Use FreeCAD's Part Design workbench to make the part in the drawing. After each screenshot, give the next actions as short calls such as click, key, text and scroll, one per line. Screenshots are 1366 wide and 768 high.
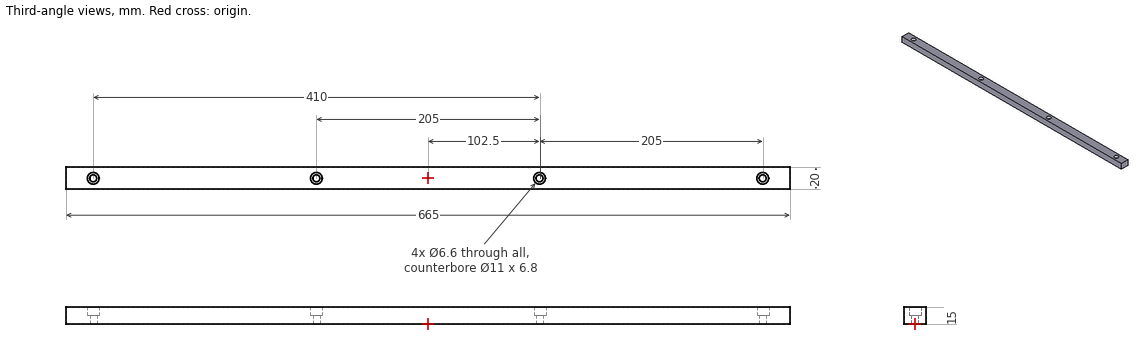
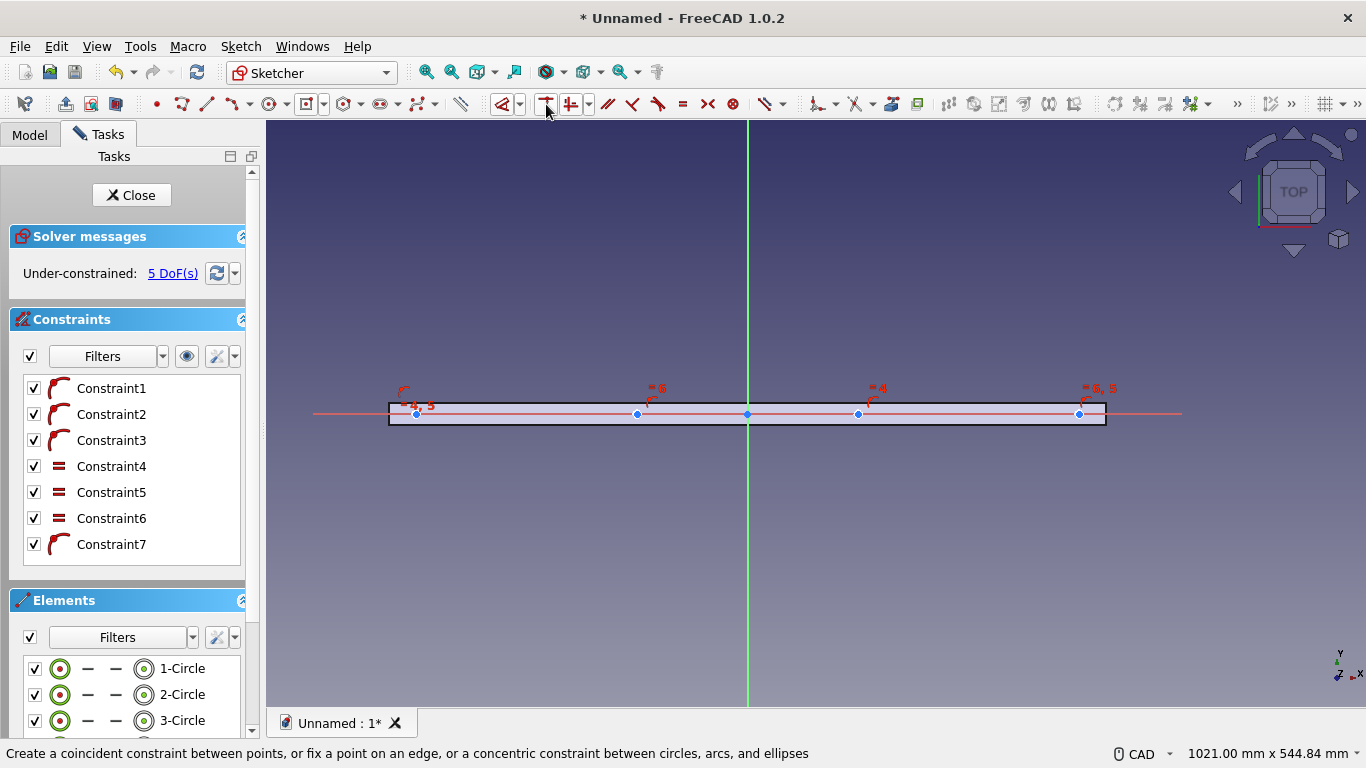
scroll(854, 414, up, 9)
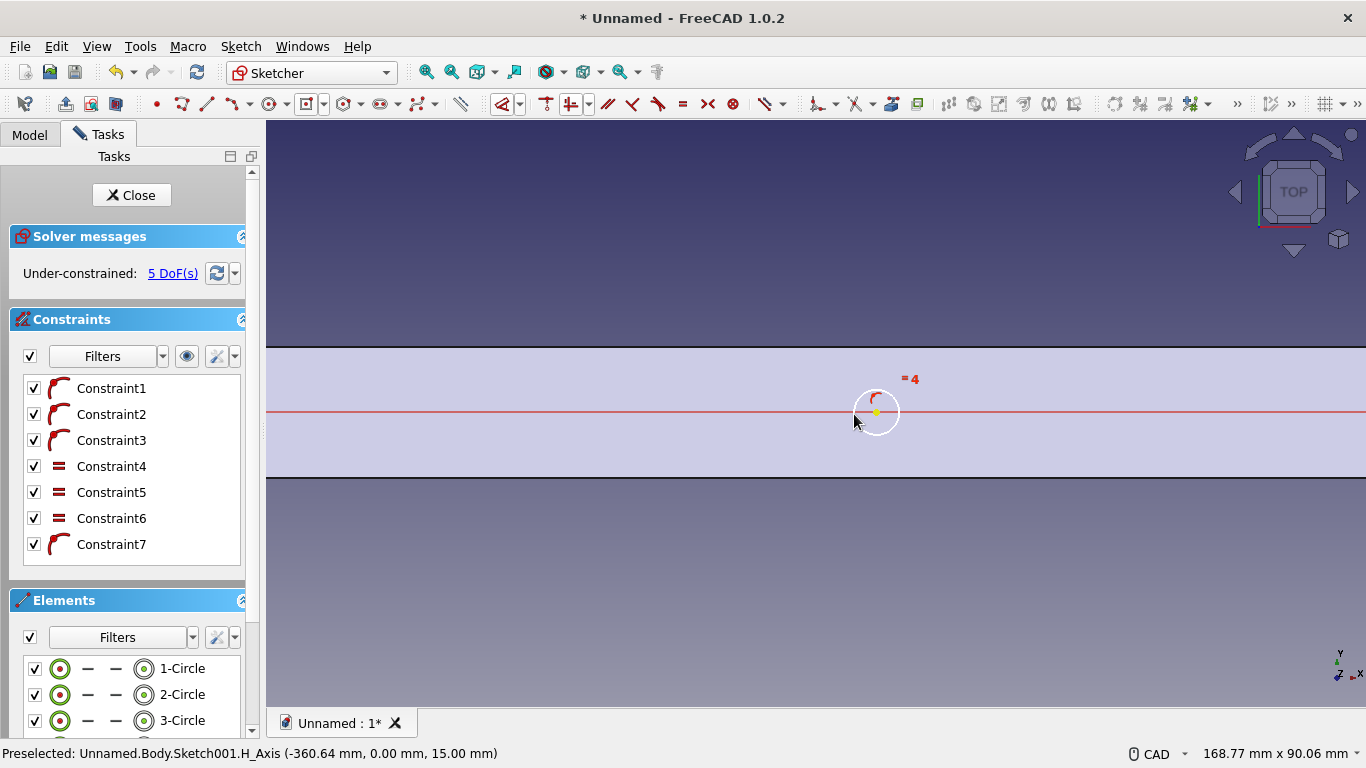
click(854, 412)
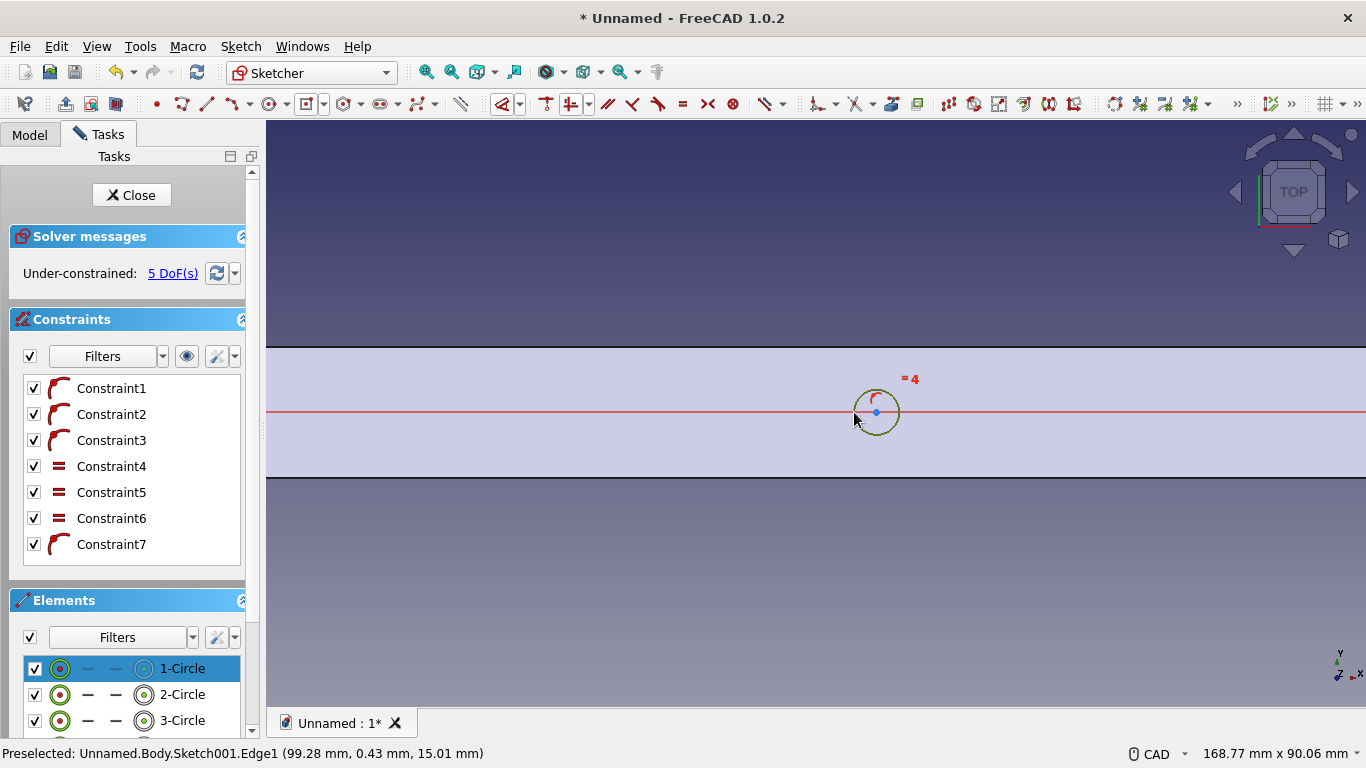
click(520, 104)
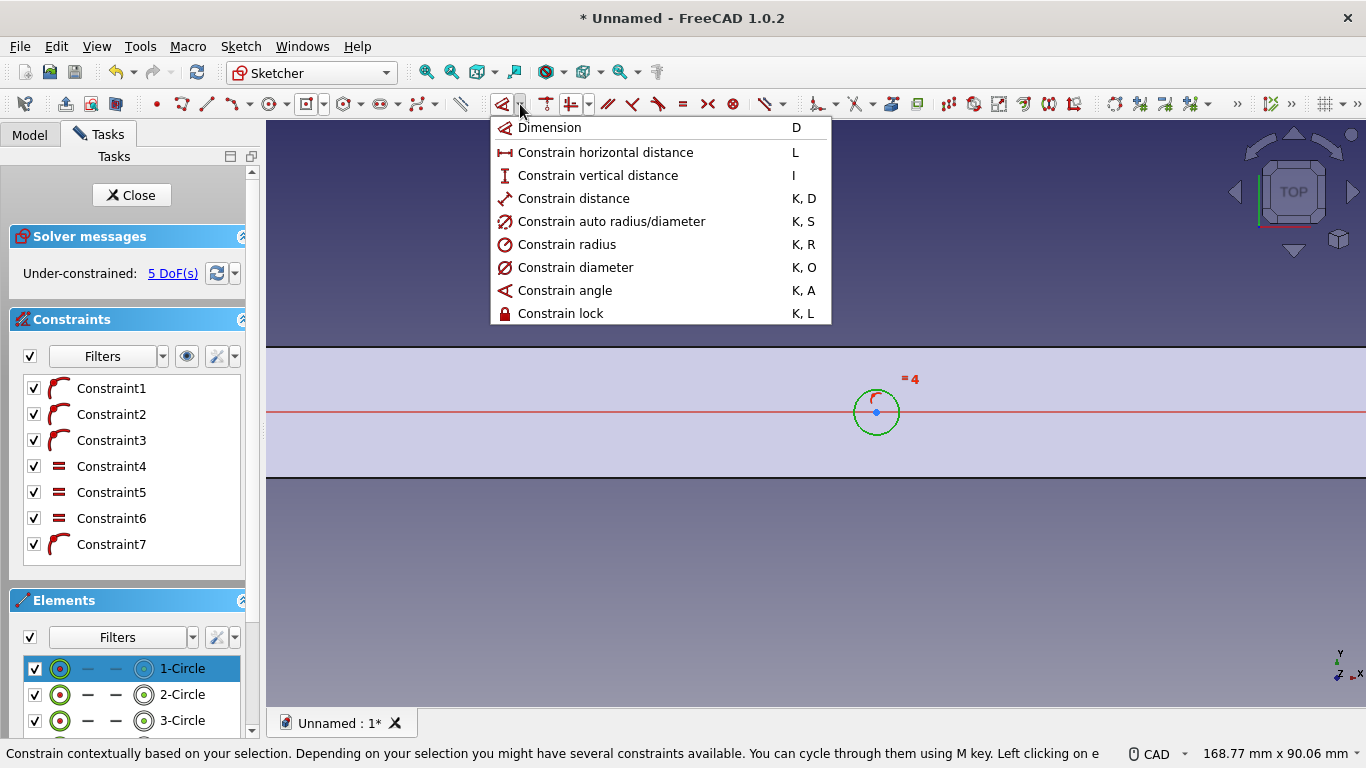
click(661, 268)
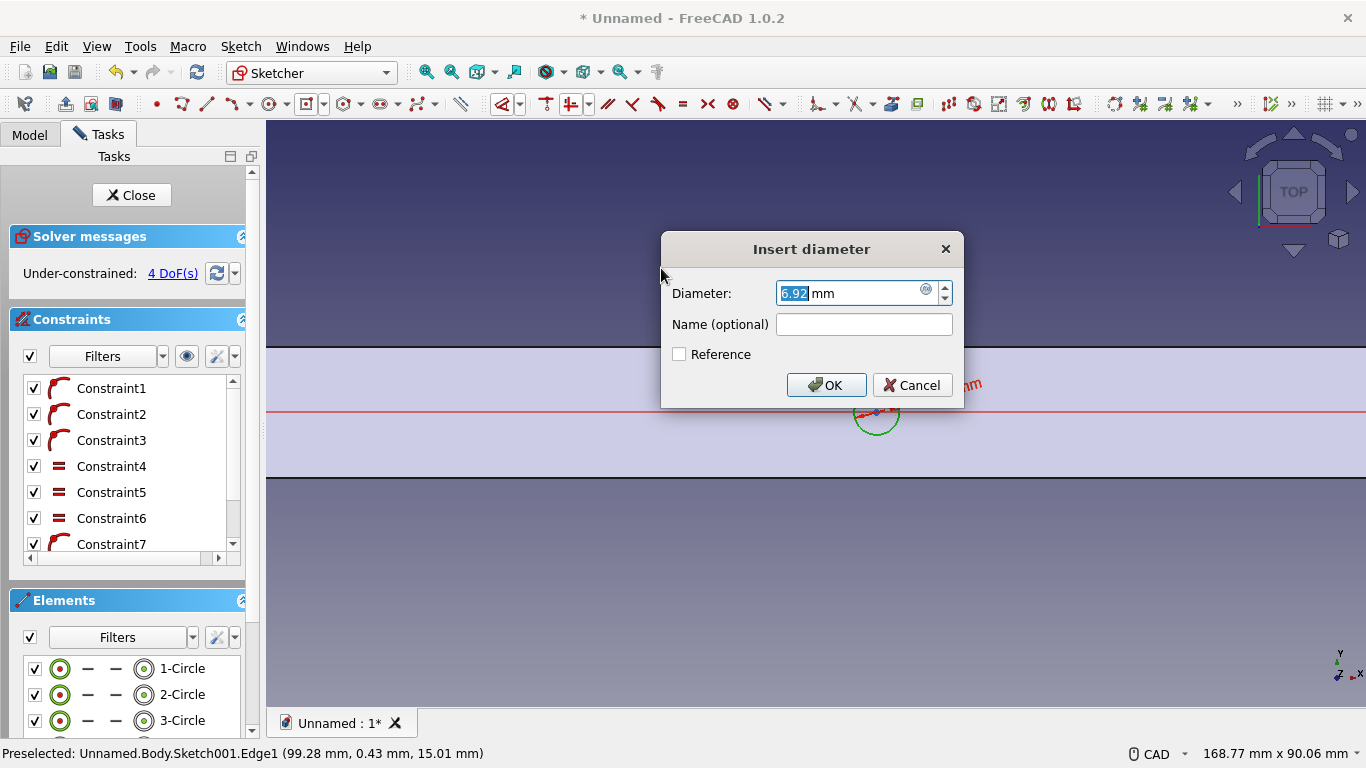
text(6.6)
key(Return)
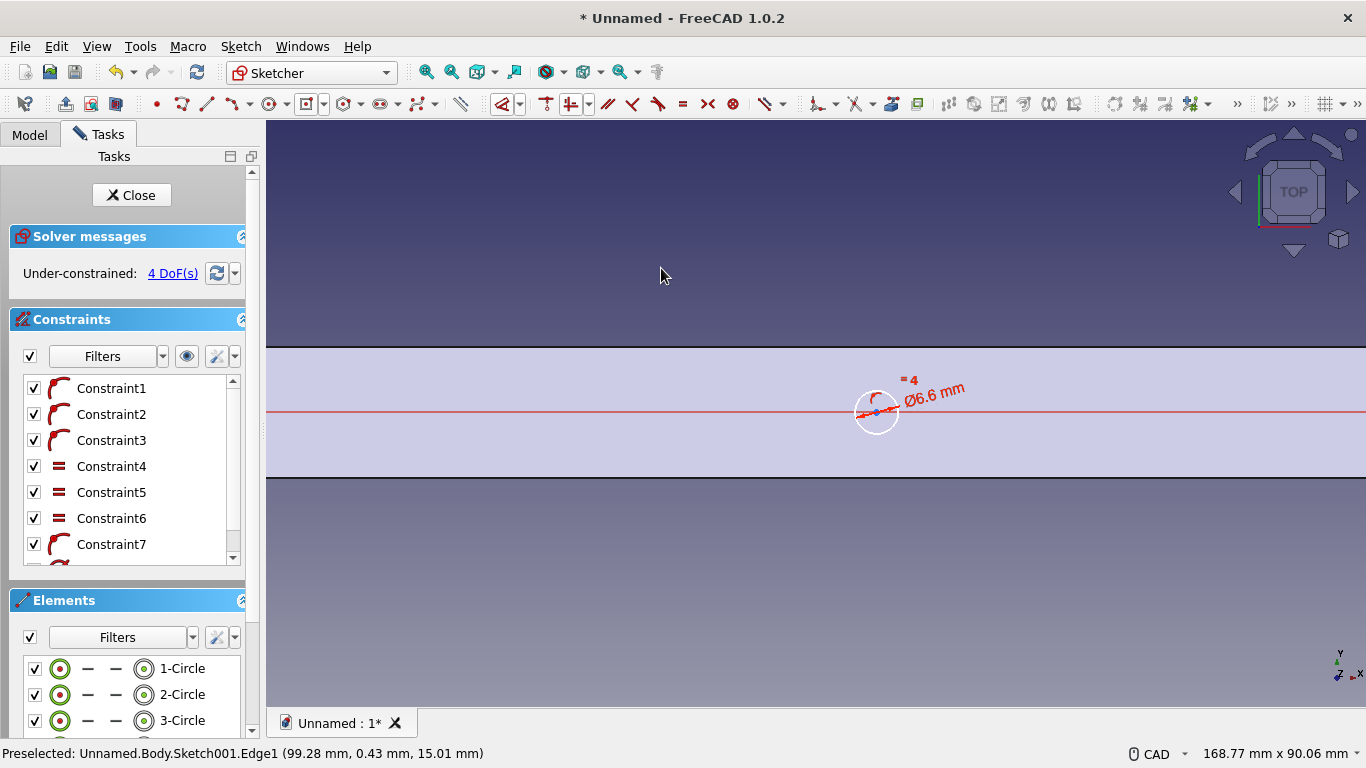
scroll(854, 414, down, 9)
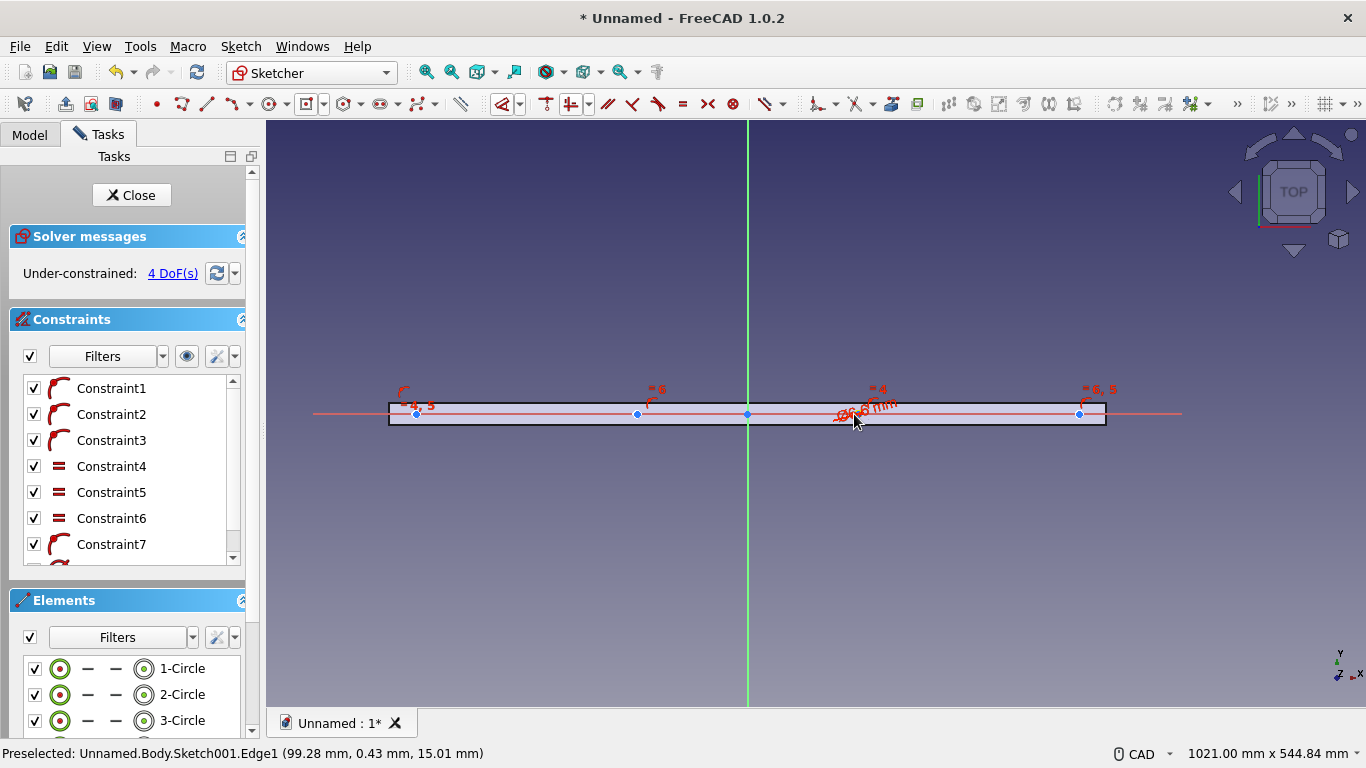
click(858, 414)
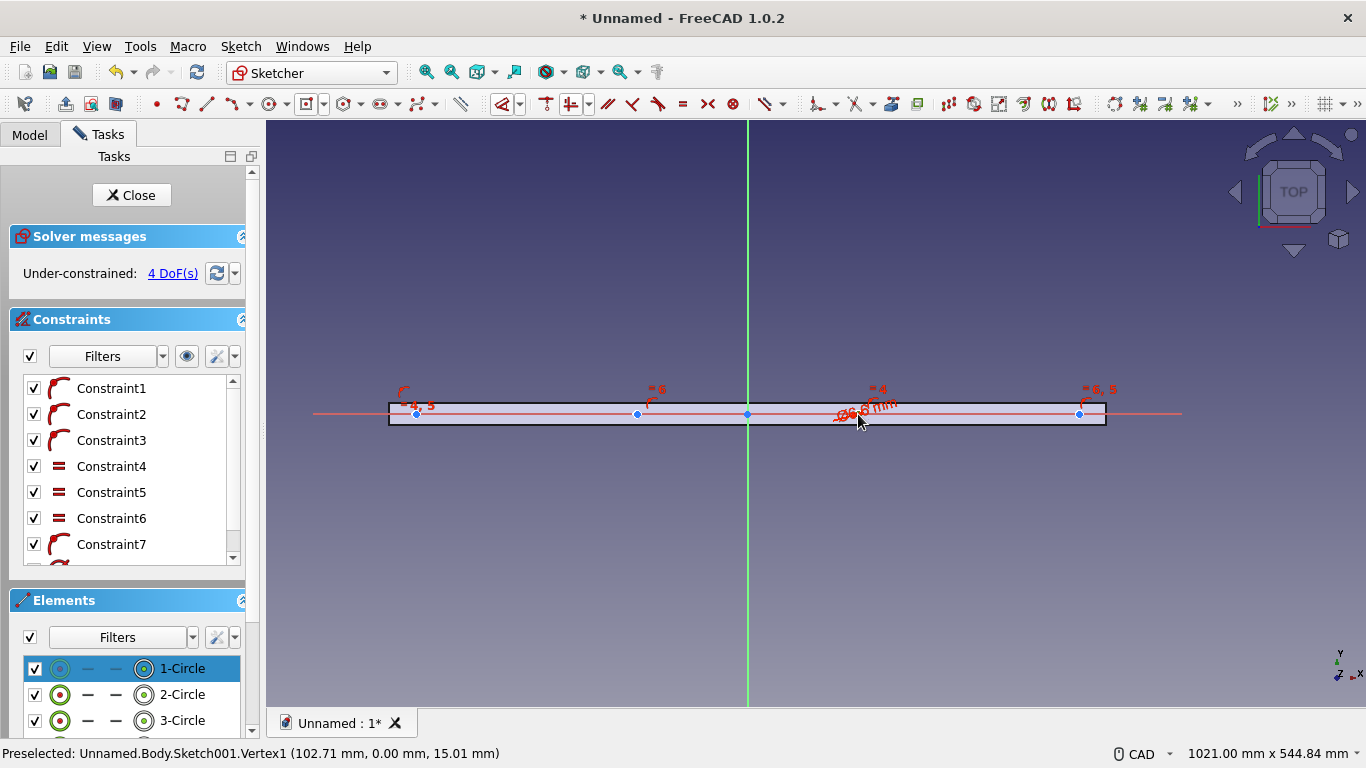
click(416, 414)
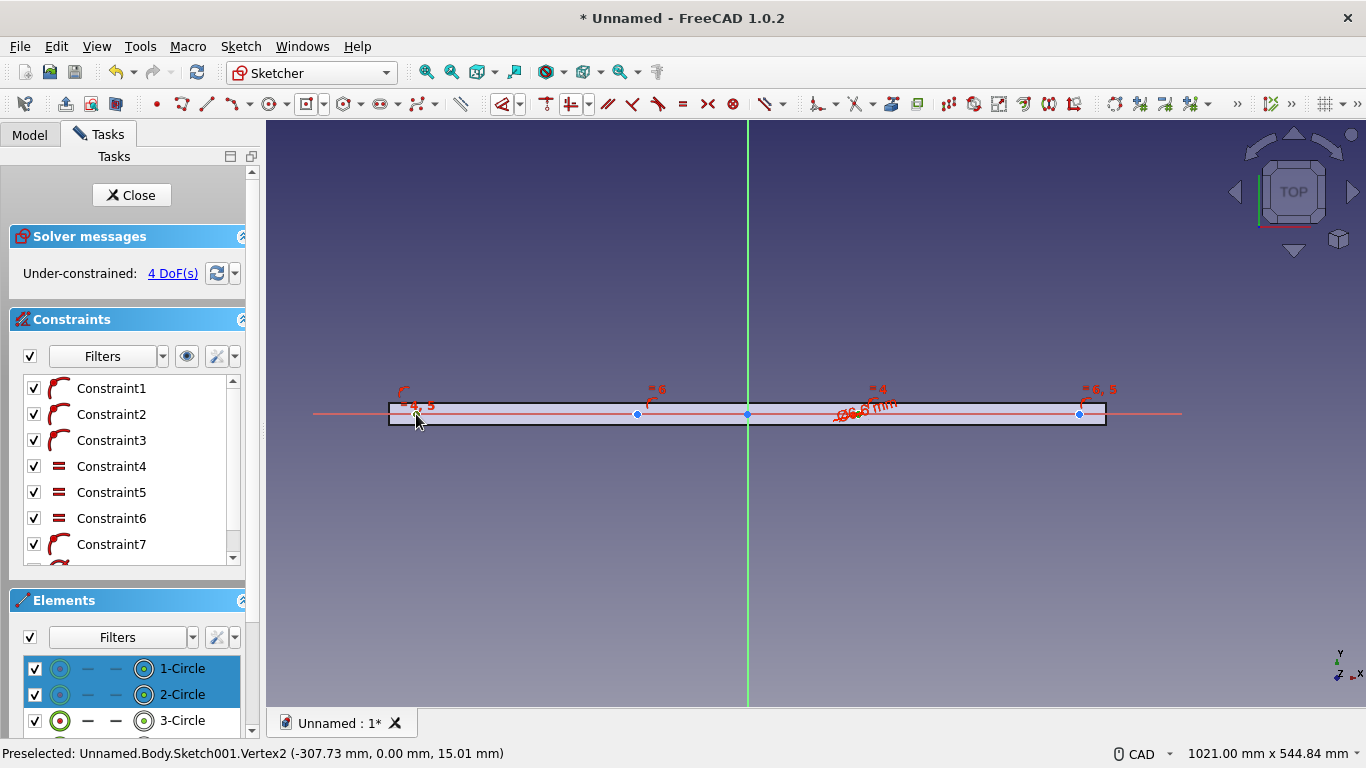
click(520, 104)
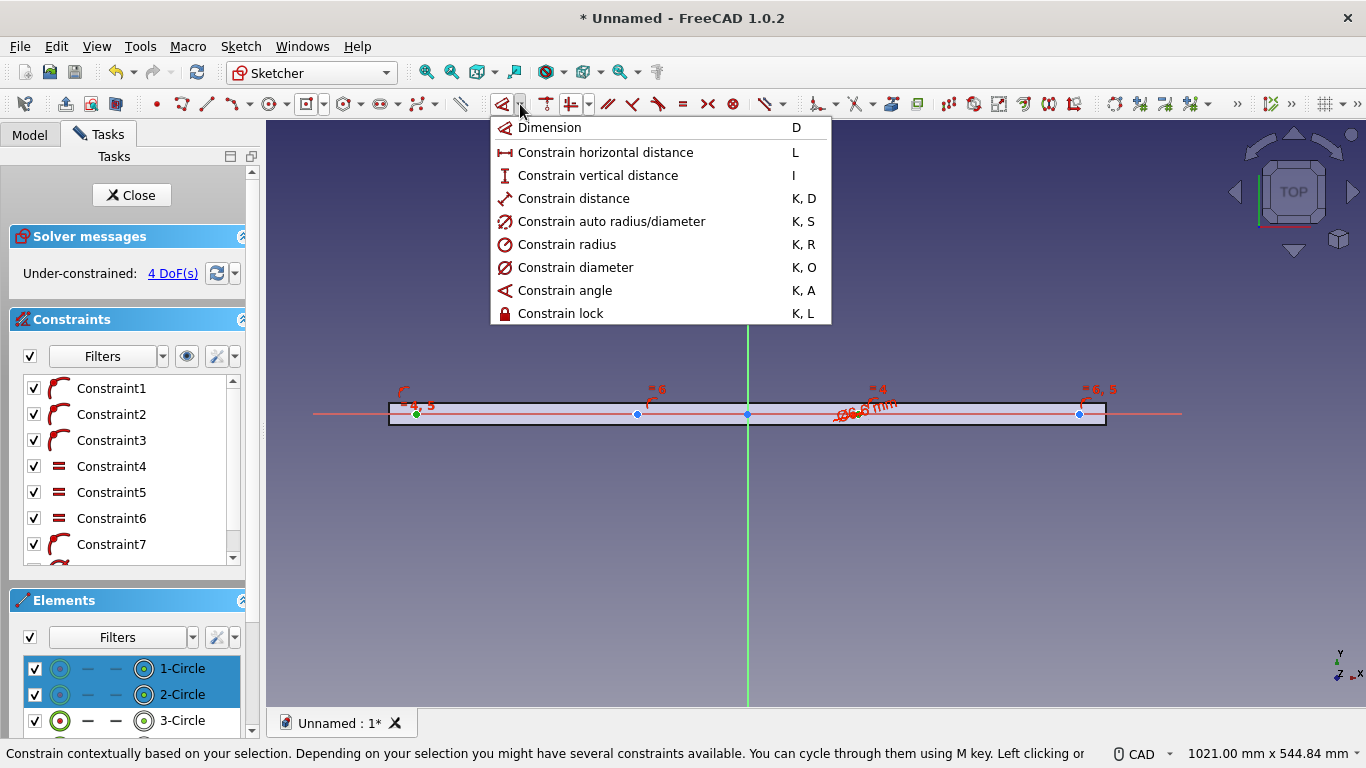
click(661, 152)